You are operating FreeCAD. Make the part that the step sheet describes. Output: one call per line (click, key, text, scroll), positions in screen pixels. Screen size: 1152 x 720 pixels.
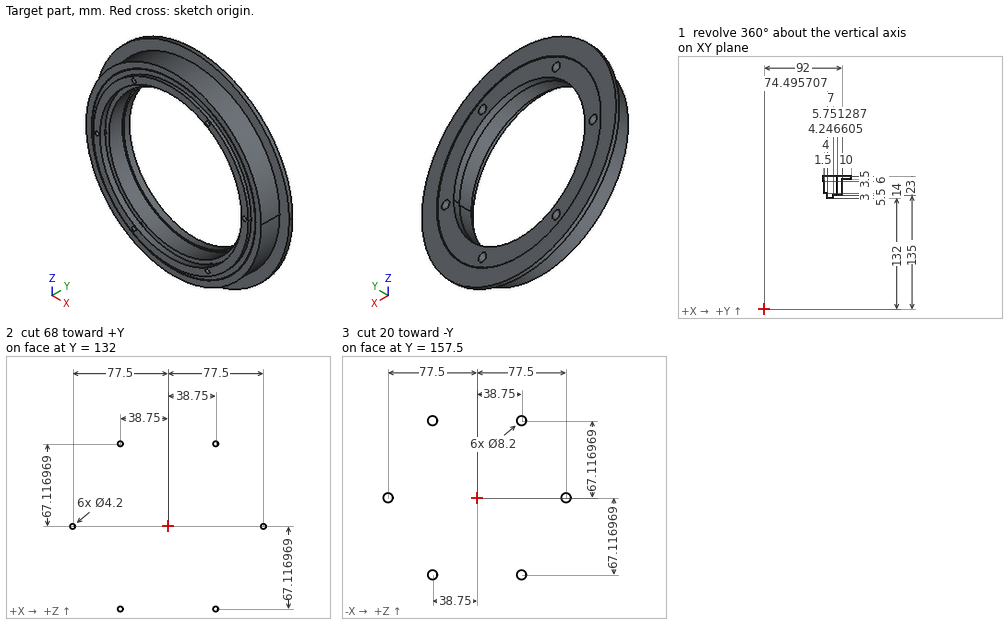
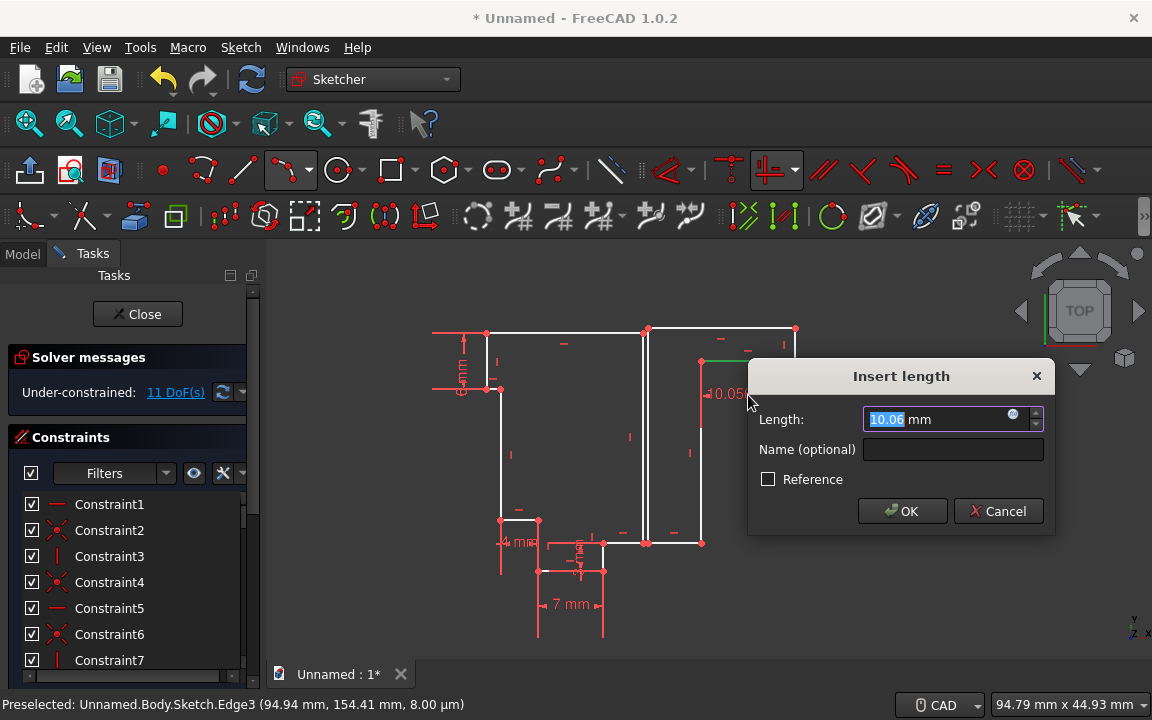
text(10)
key(Return)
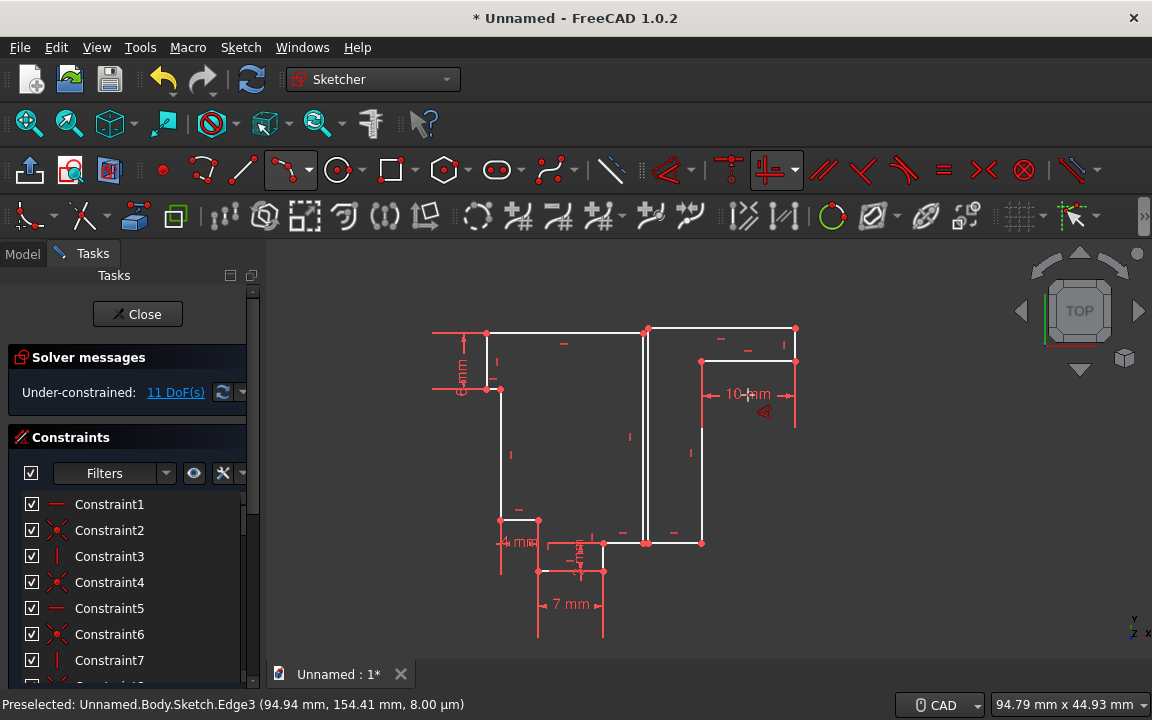
scroll(648, 393, up, 5)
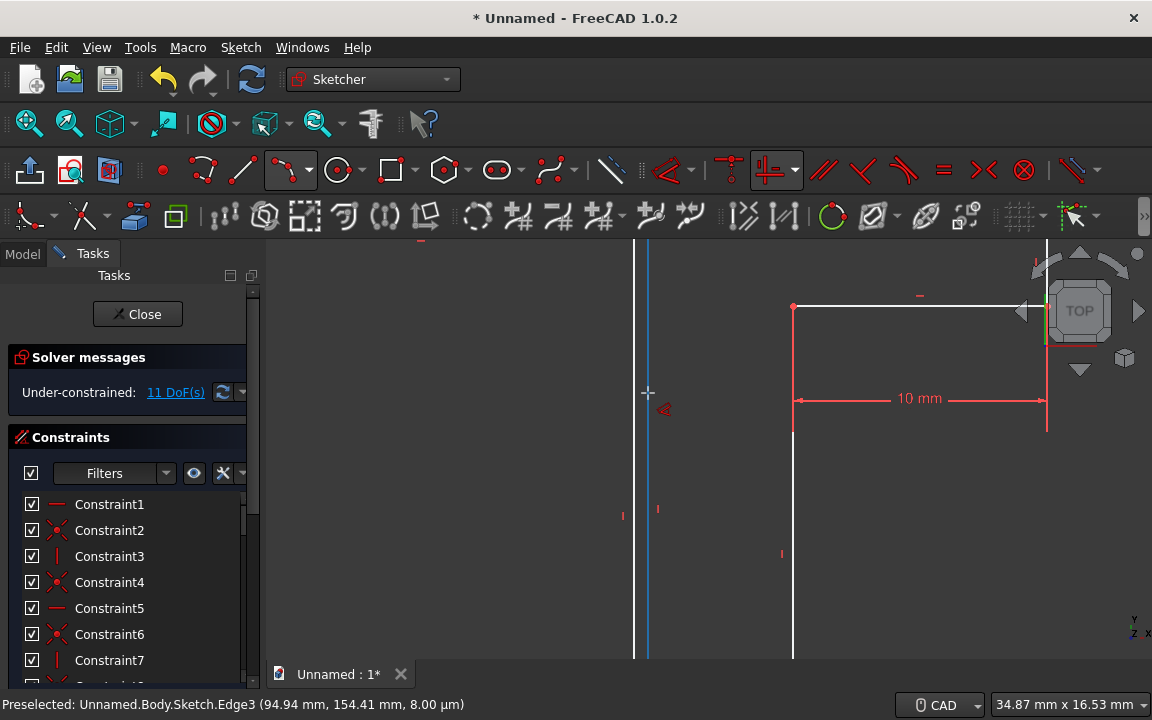
click(648, 392)
click(682, 449)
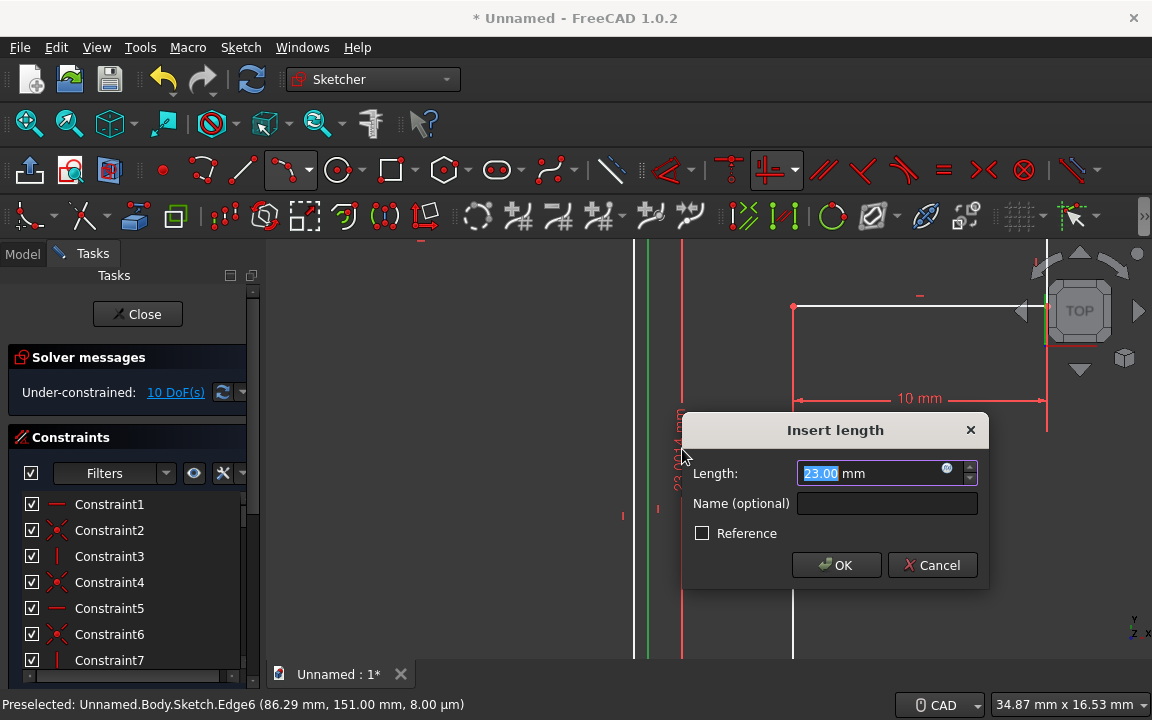
text(23)
key(Return)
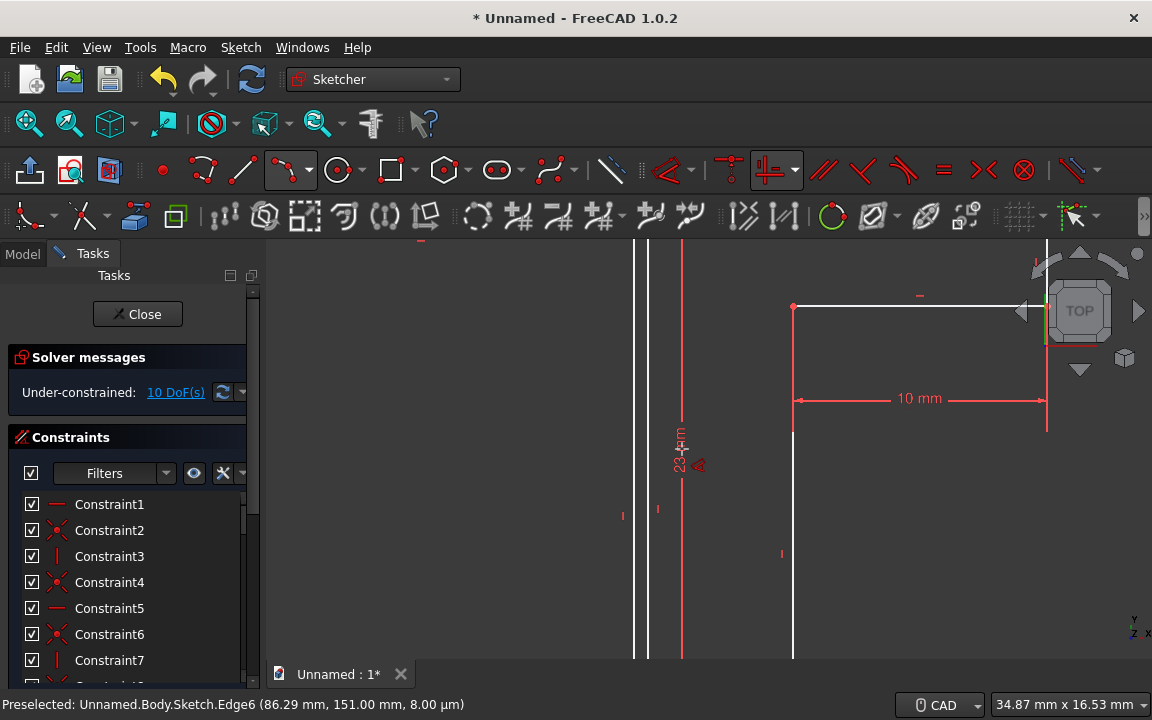
scroll(648, 393, down, 5)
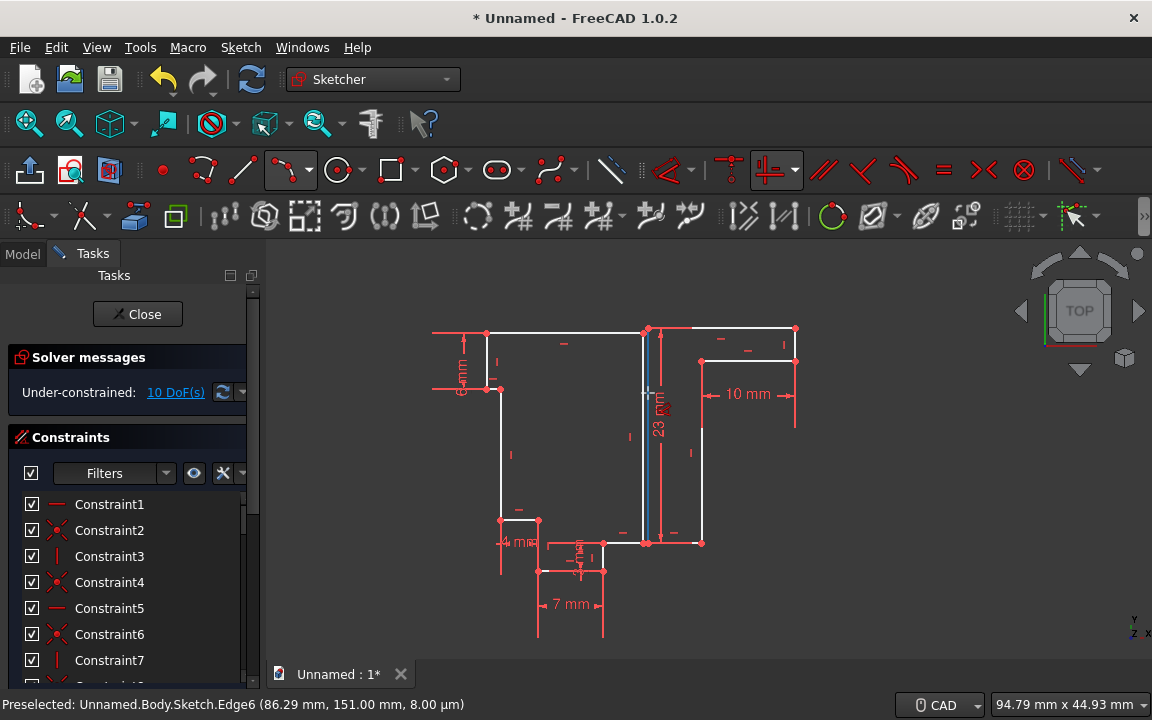
click(501, 429)
click(467, 455)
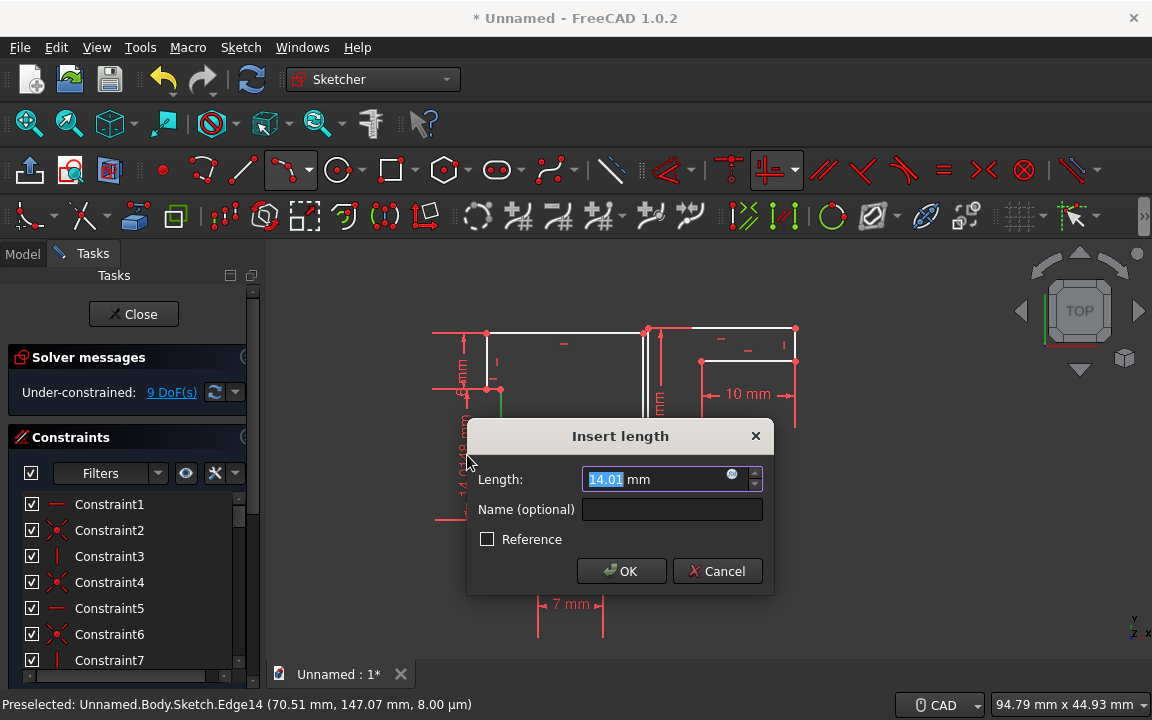
text(14)
key(Return)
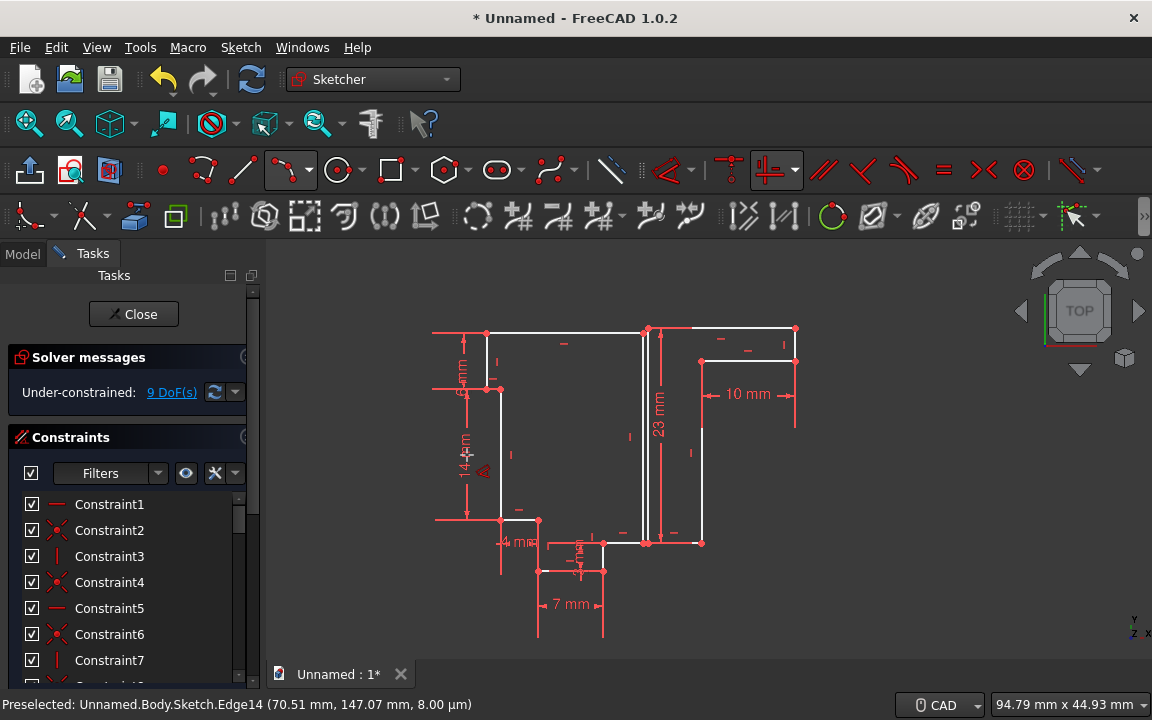
scroll(795, 351, up, 2)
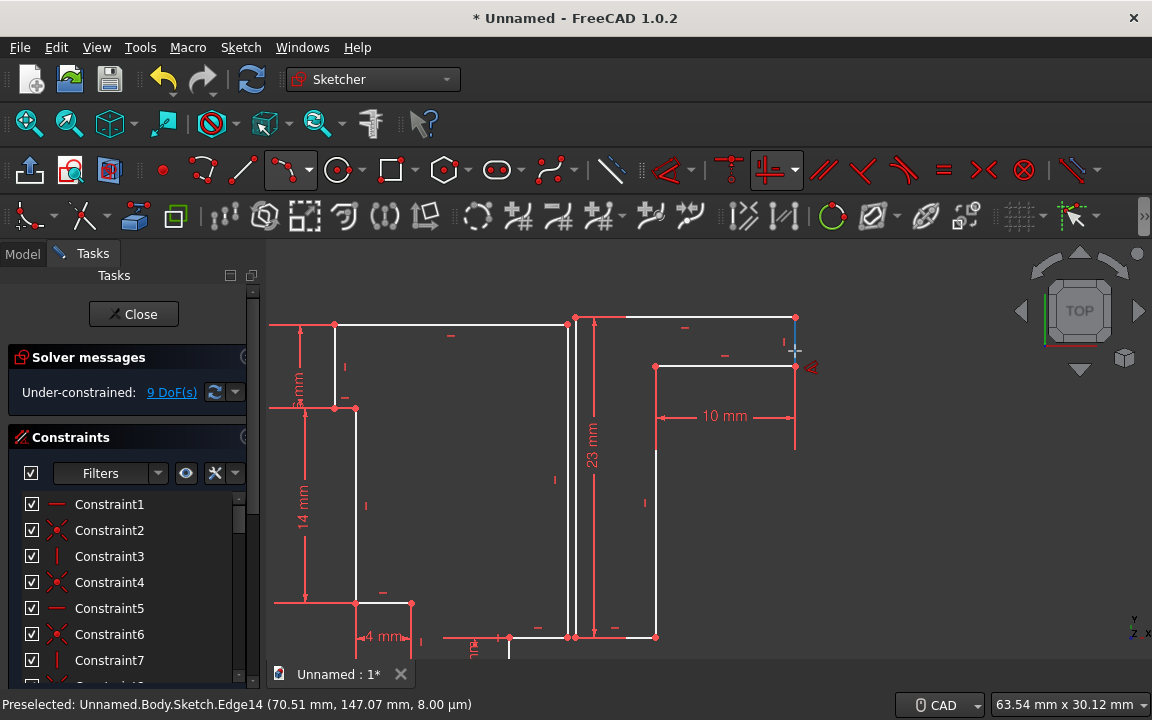
click(795, 352)
click(829, 342)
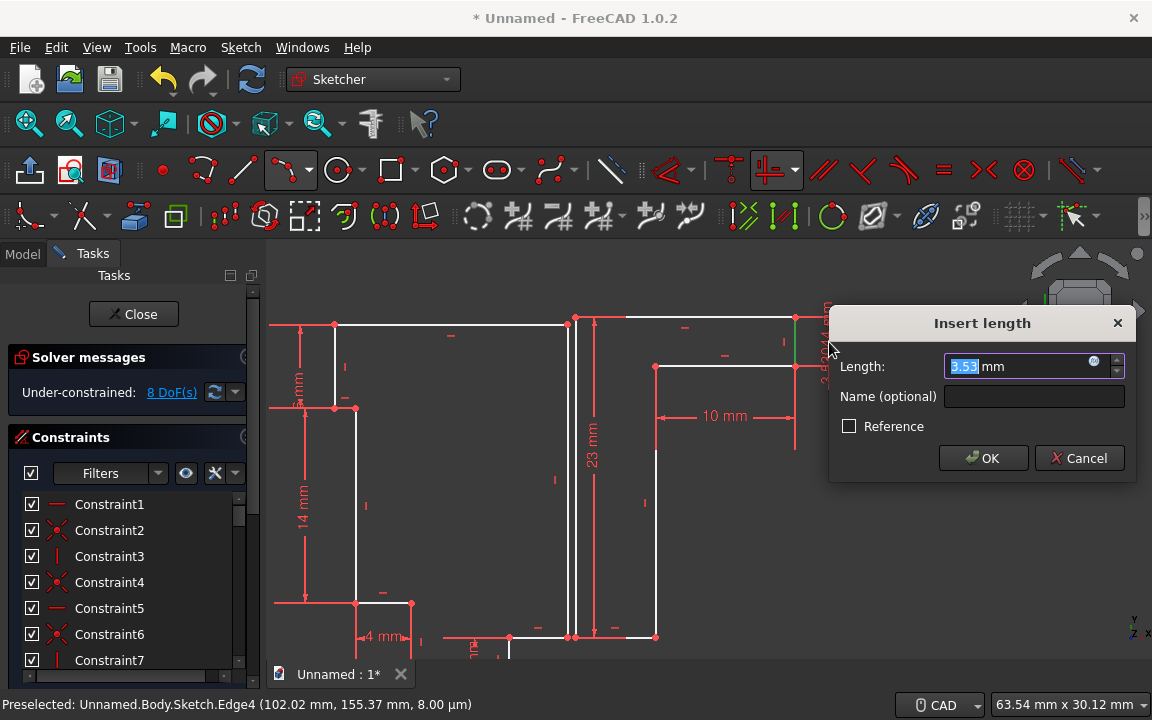
text(3.5)
key(Return)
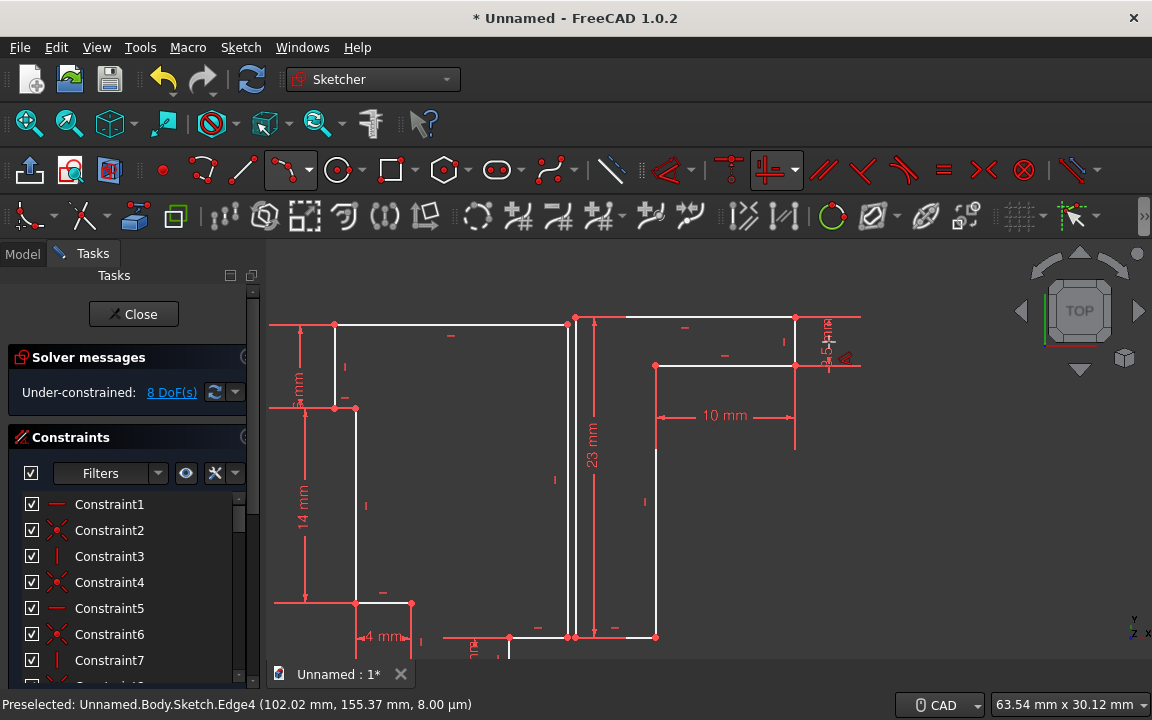
scroll(345, 408, up, 4)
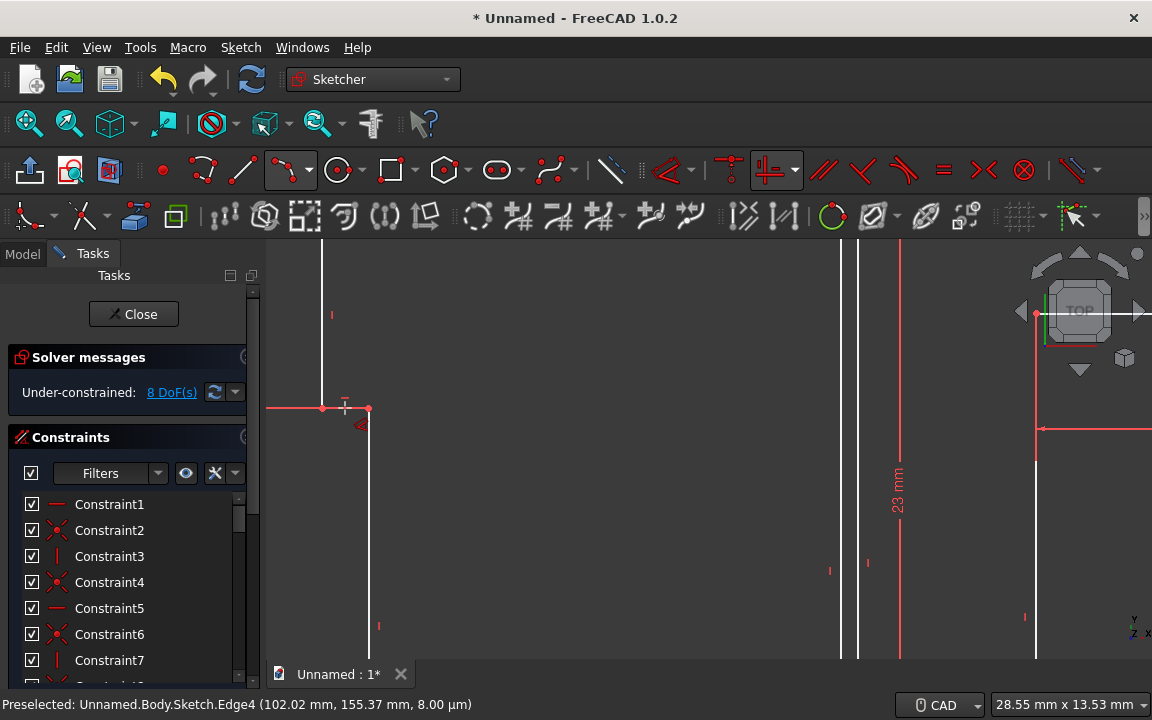
click(345, 408)
click(345, 374)